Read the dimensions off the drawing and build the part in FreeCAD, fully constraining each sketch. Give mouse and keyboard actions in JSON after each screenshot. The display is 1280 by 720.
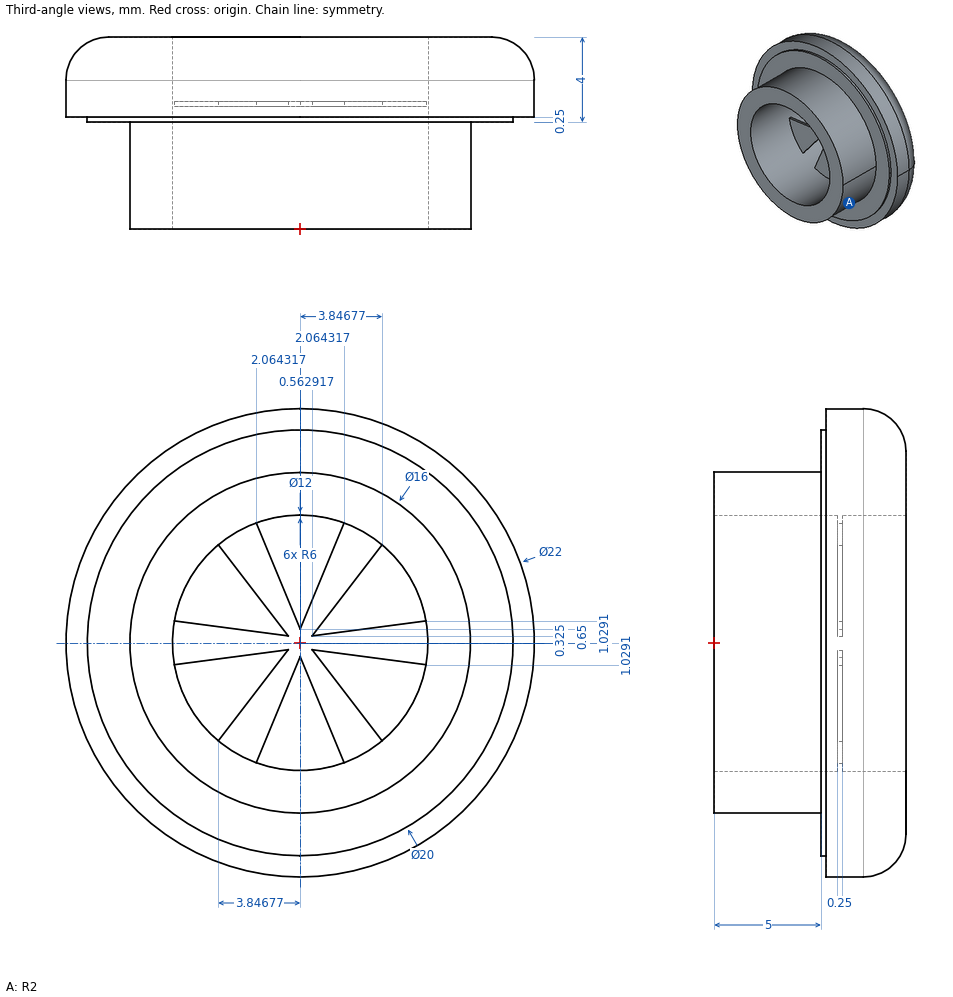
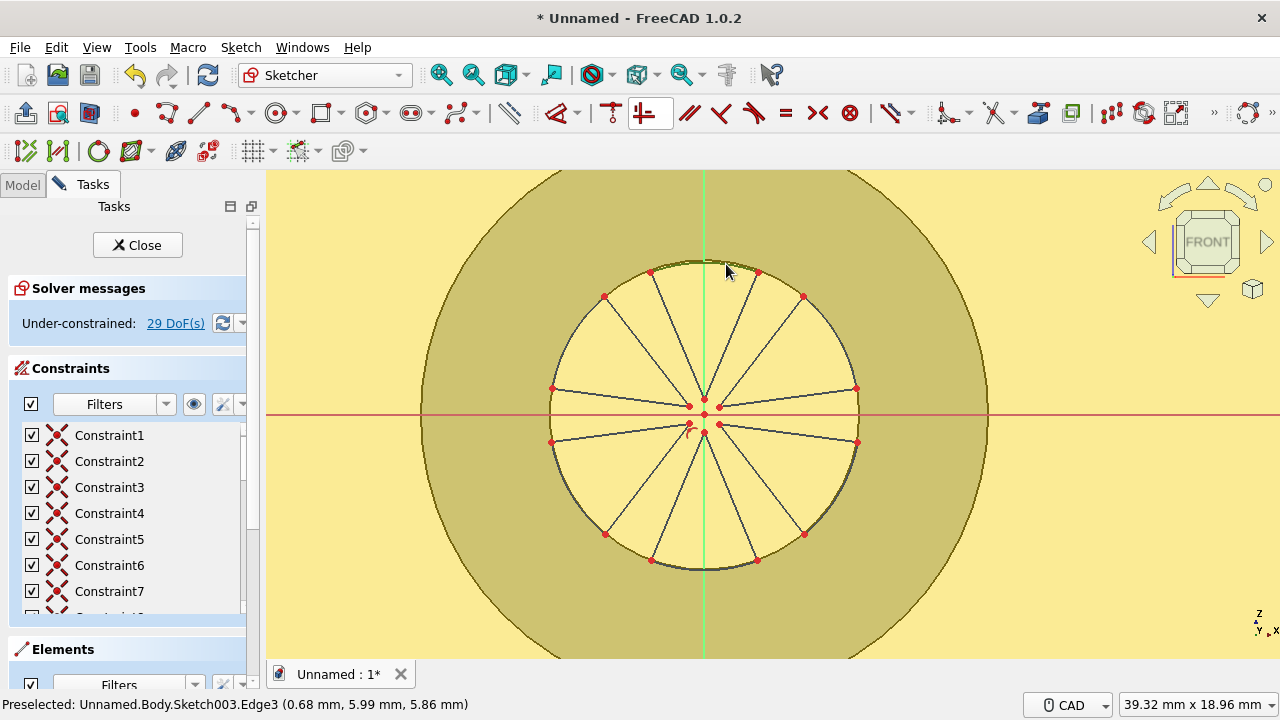
{"action": "left_click", "coordinate": [848, 358]}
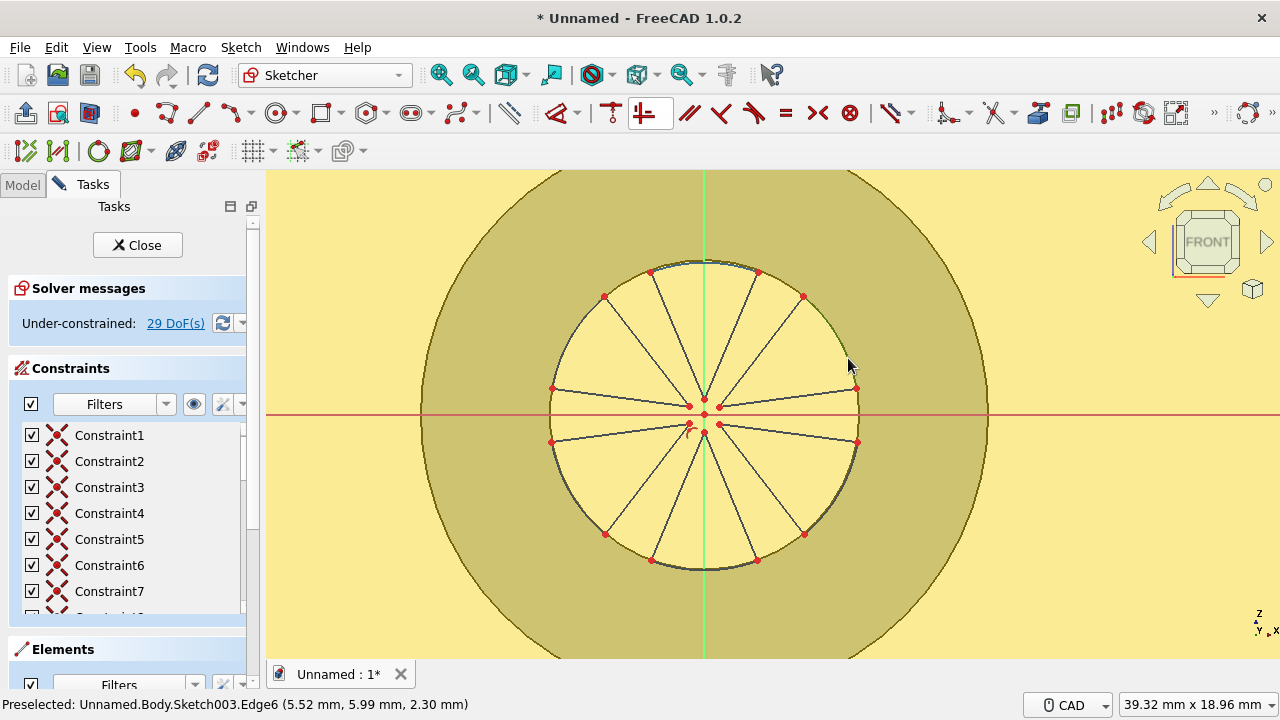
{"action": "left_click", "coordinate": [827, 511]}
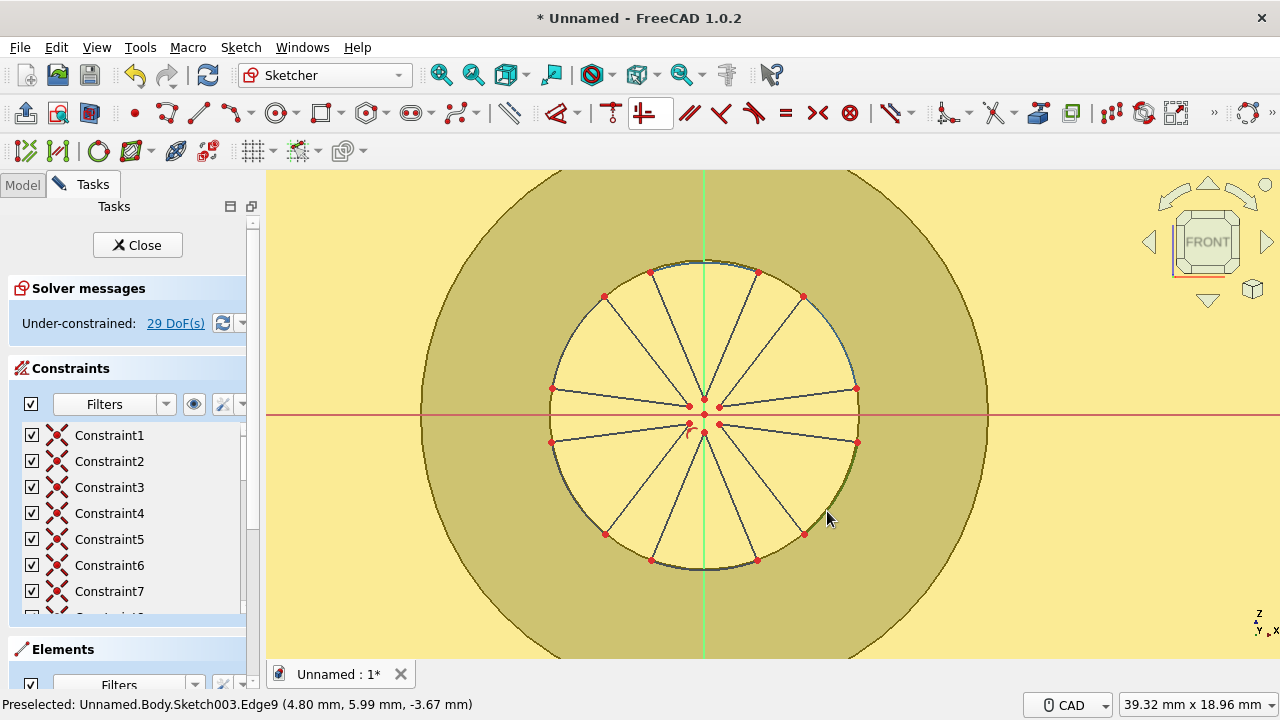
{"action": "left_click", "coordinate": [683, 569]}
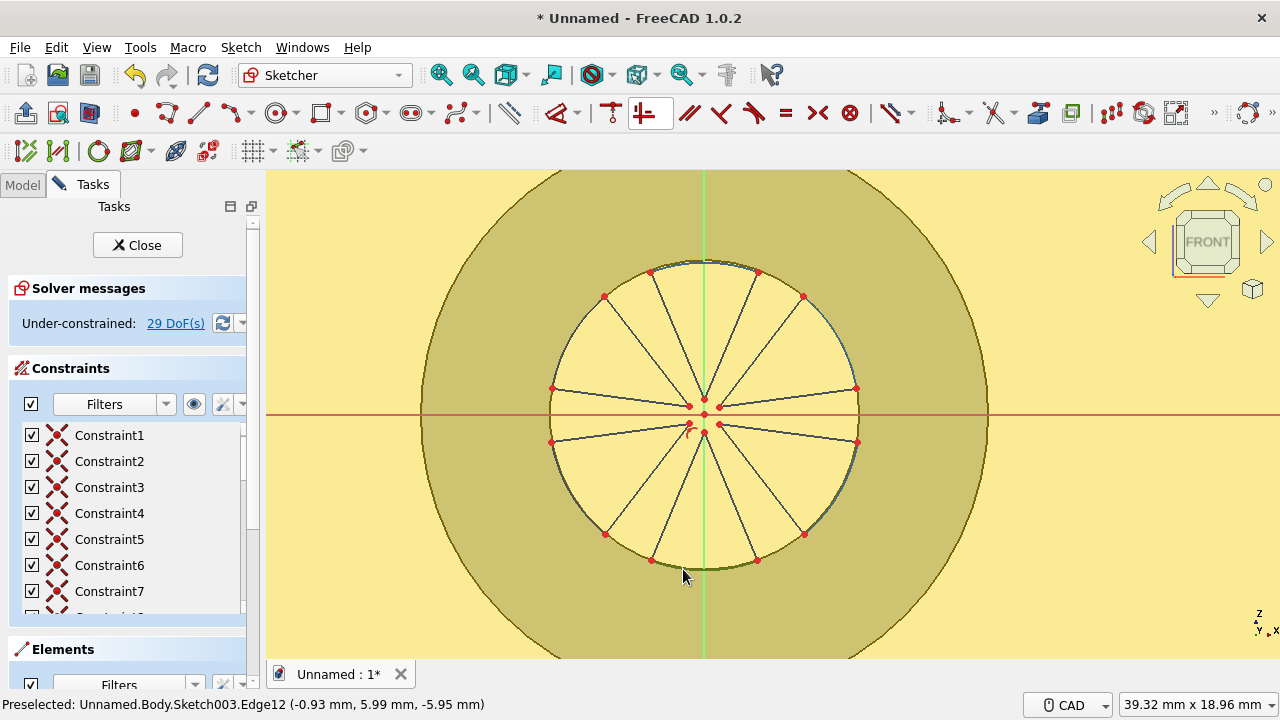
{"action": "left_click", "coordinate": [561, 473]}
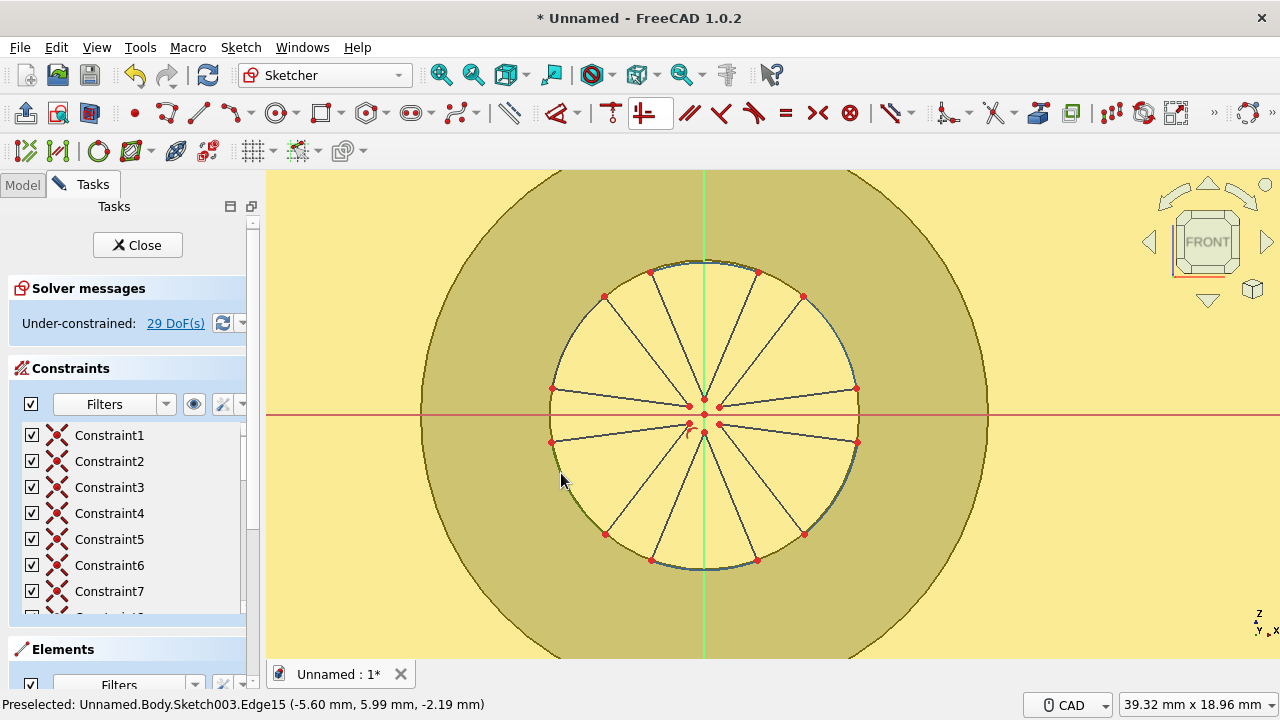
{"action": "left_click", "coordinate": [583, 320]}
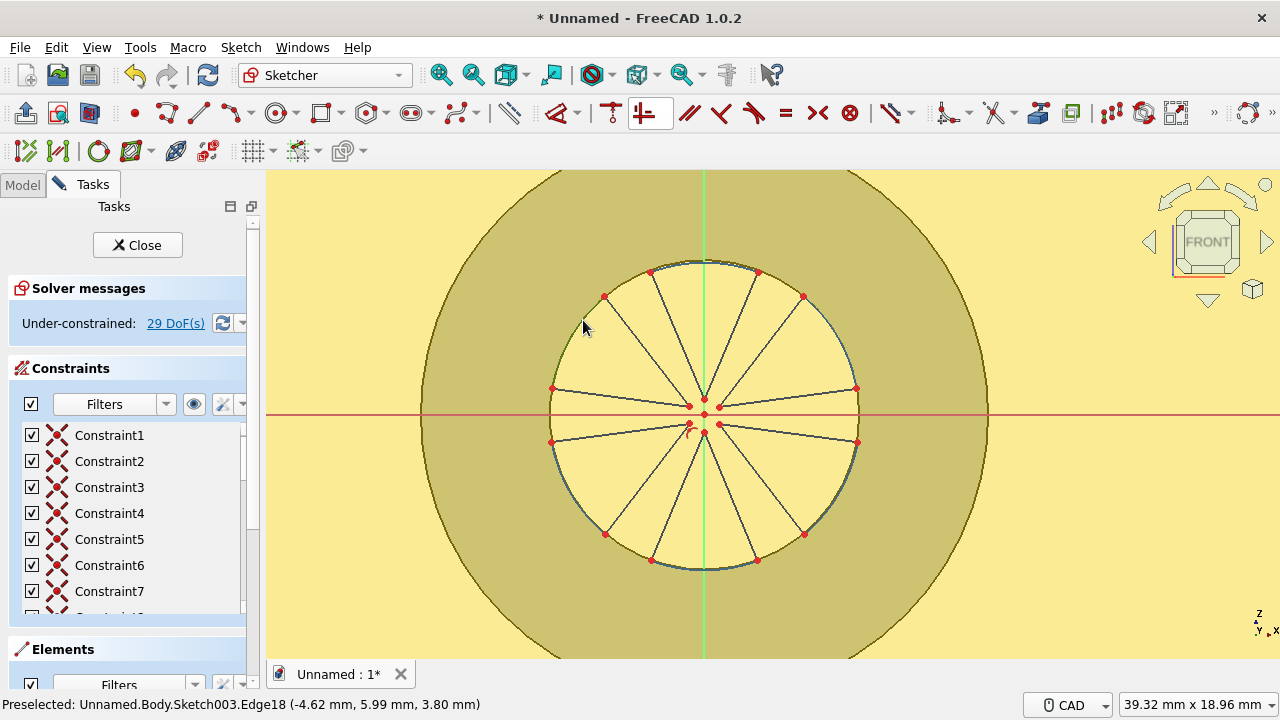
{"action": "key", "text": "e"}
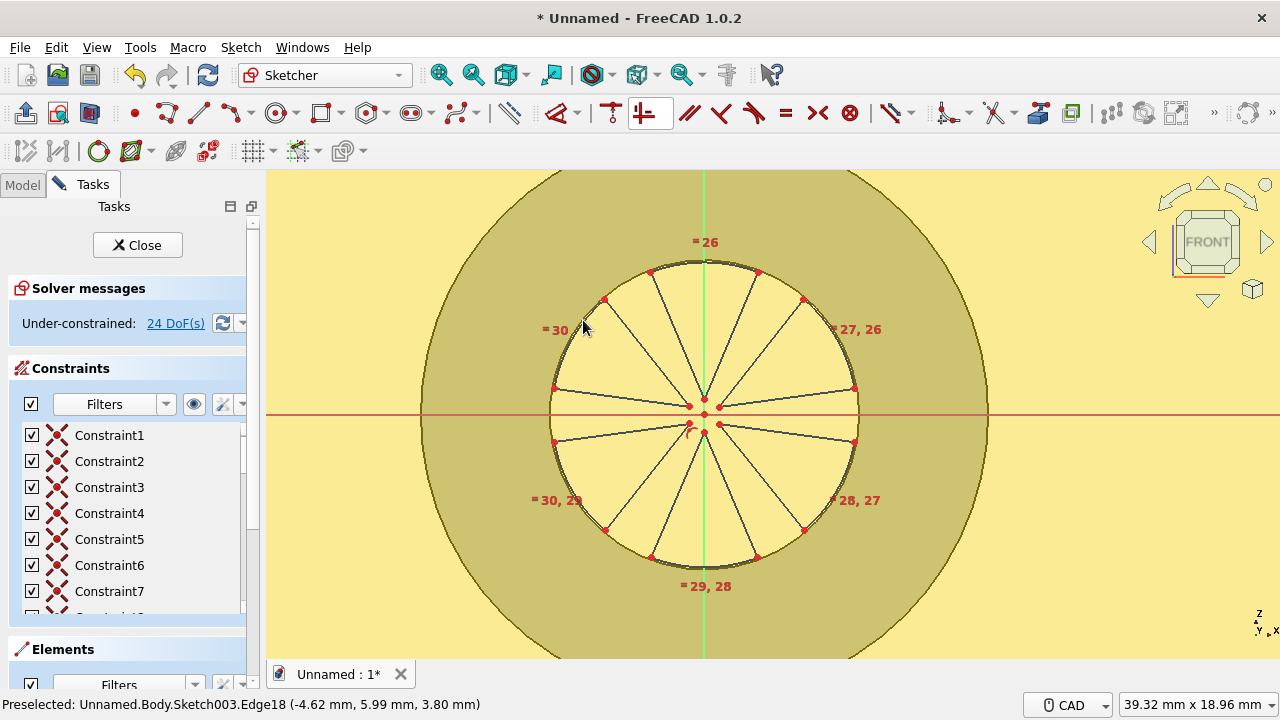
{"action": "left_click", "coordinate": [719, 407]}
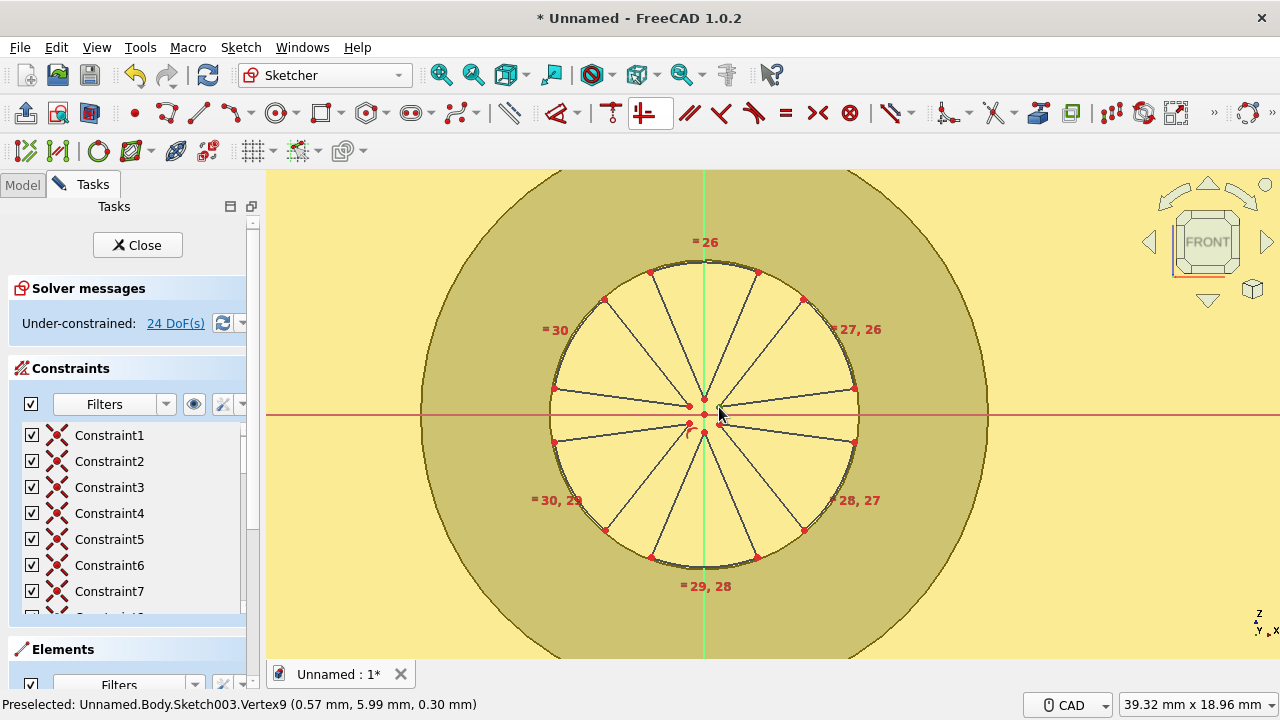
{"action": "left_click", "coordinate": [719, 424]}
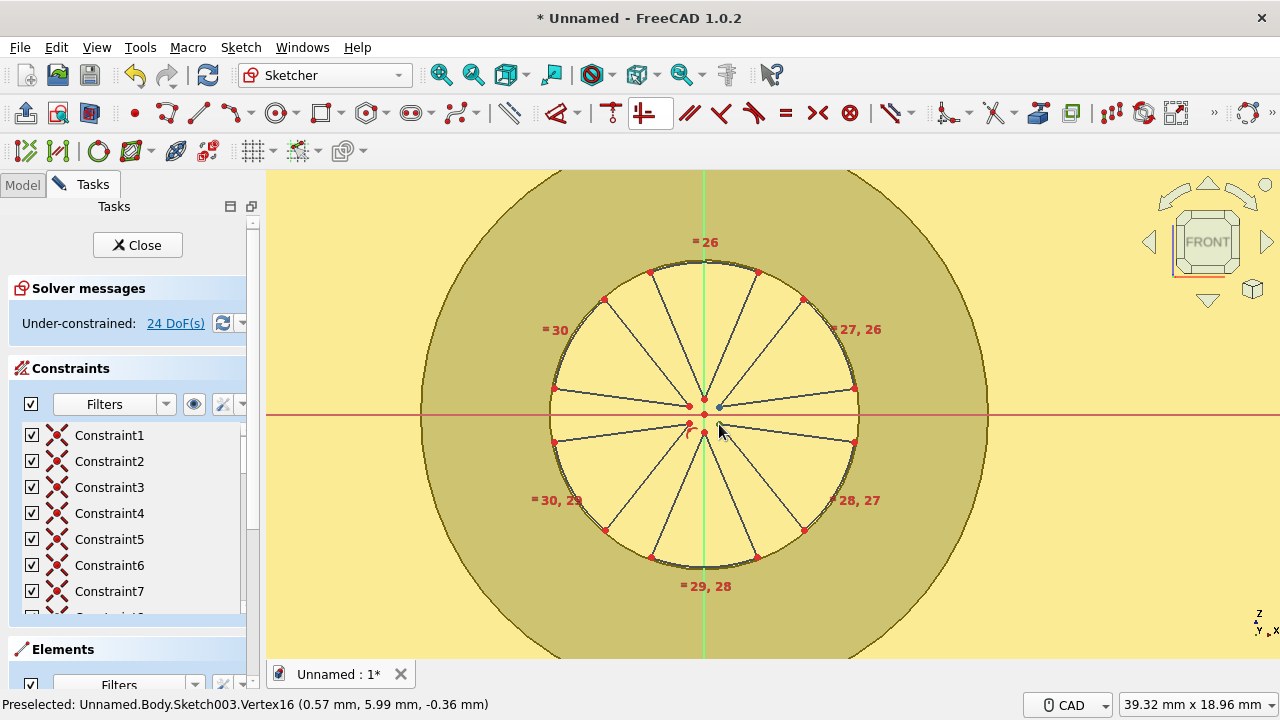
{"action": "left_click", "coordinate": [353, 415]}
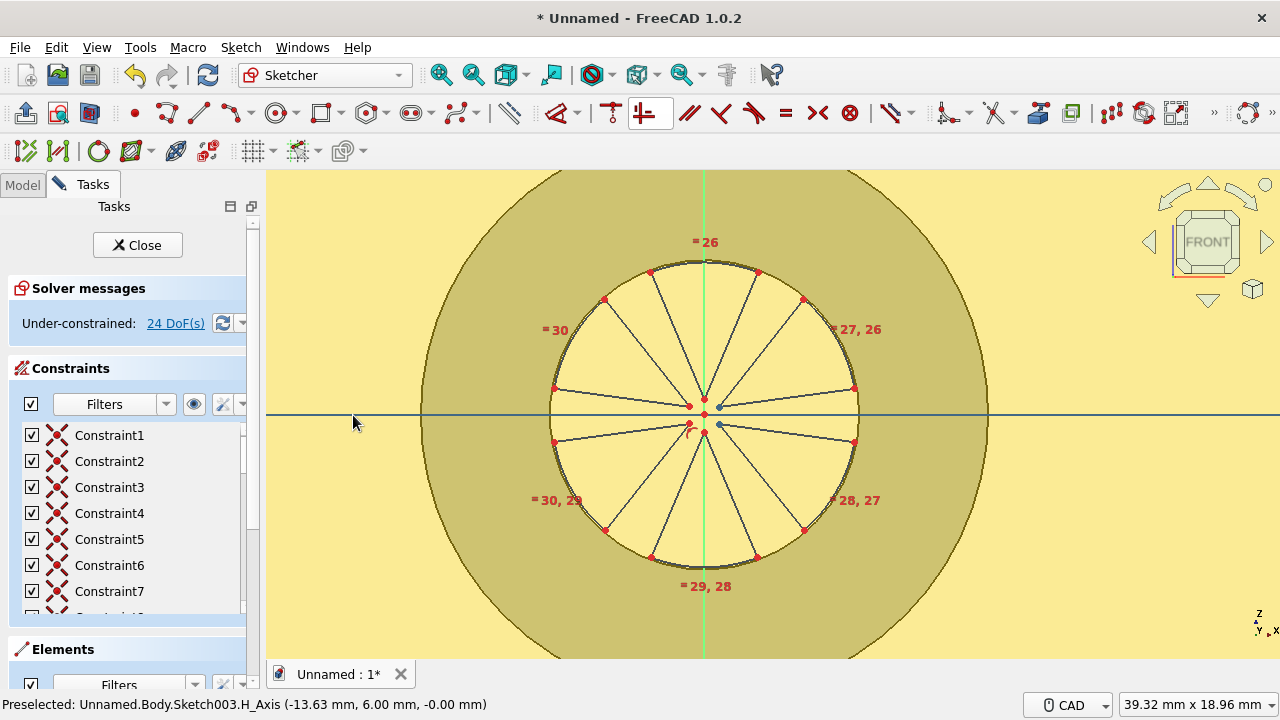
{"action": "key", "text": "s"}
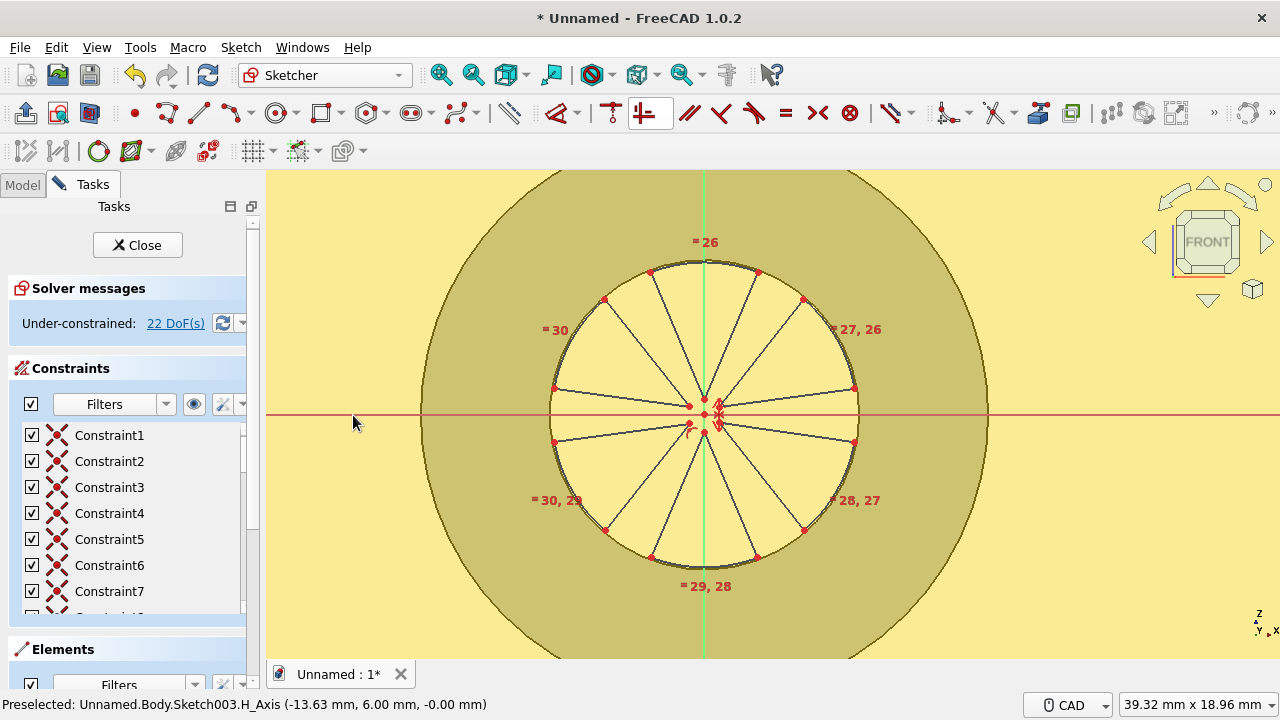
{"action": "left_click", "coordinate": [705, 400]}